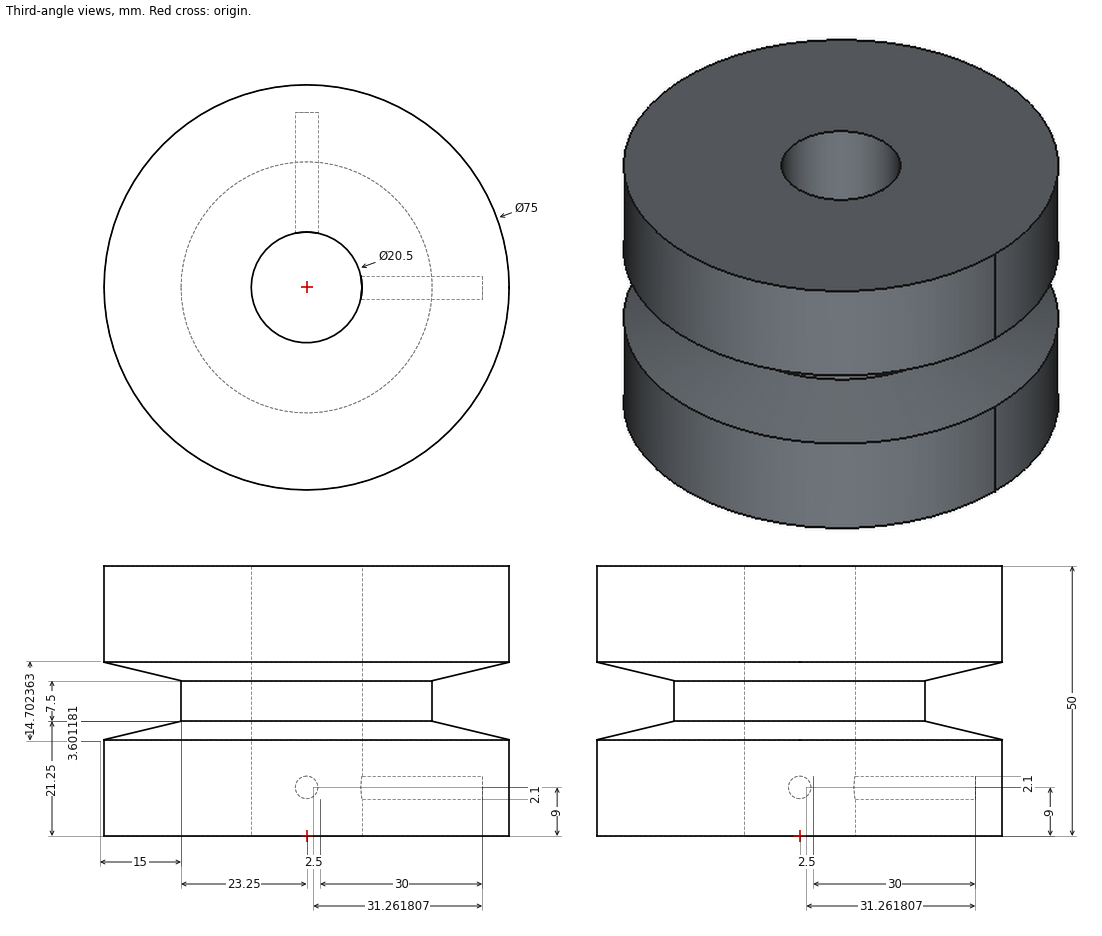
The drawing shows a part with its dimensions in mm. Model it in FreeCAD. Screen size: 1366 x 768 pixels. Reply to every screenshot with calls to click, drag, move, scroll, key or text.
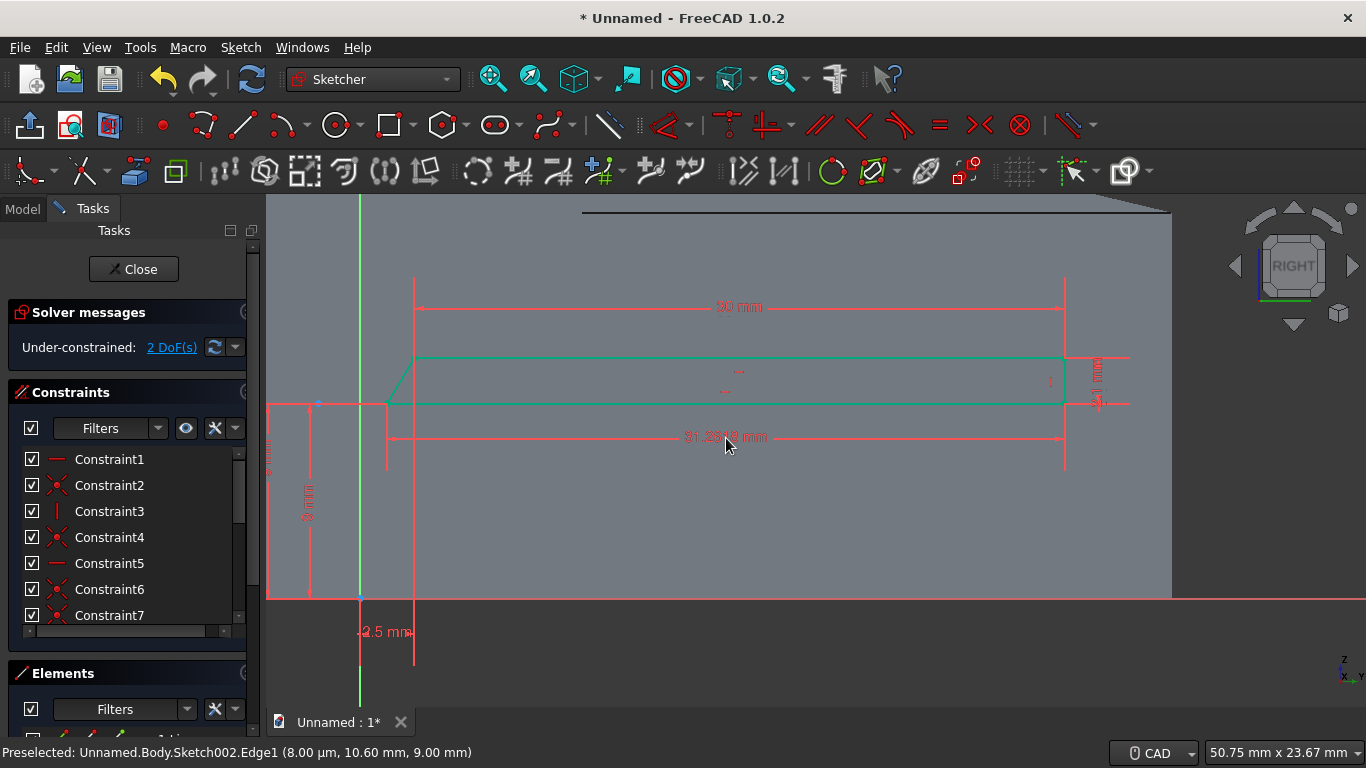
click(134, 269)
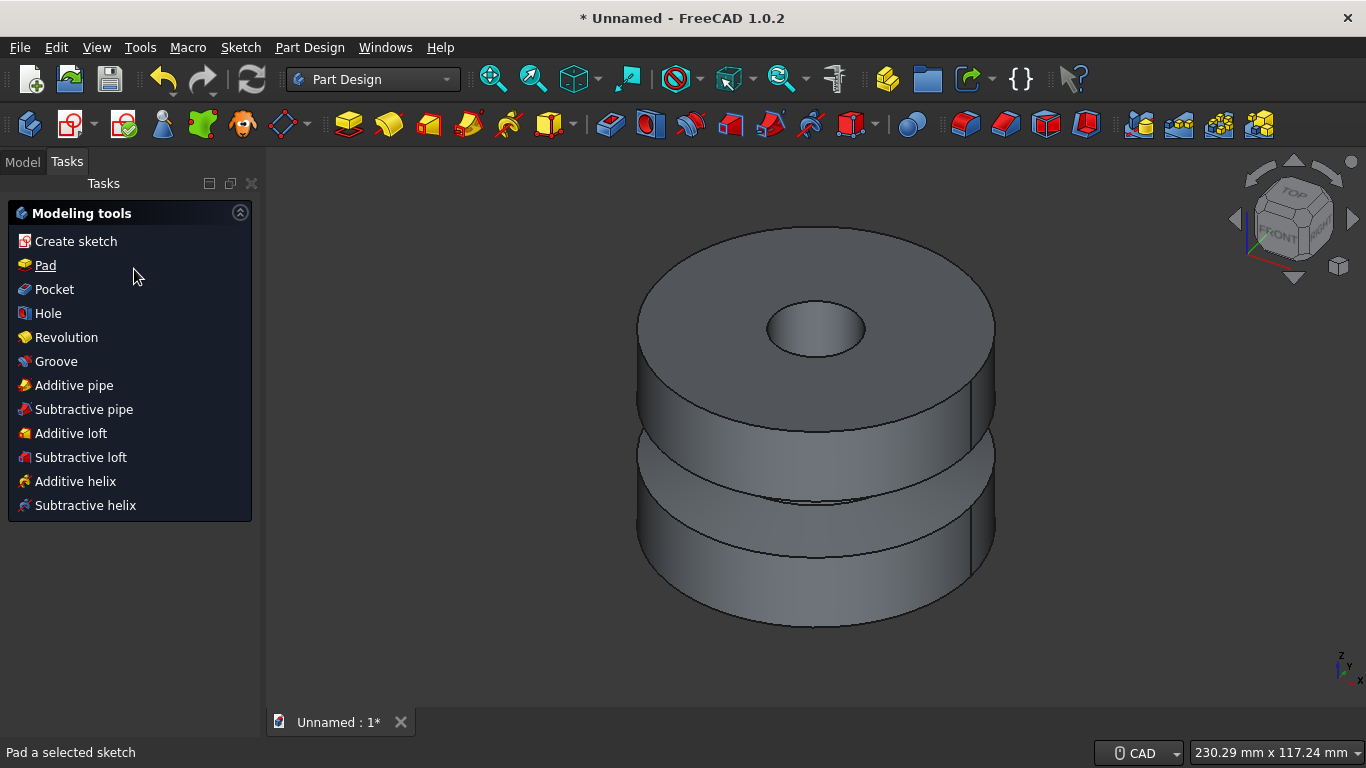
click(692, 124)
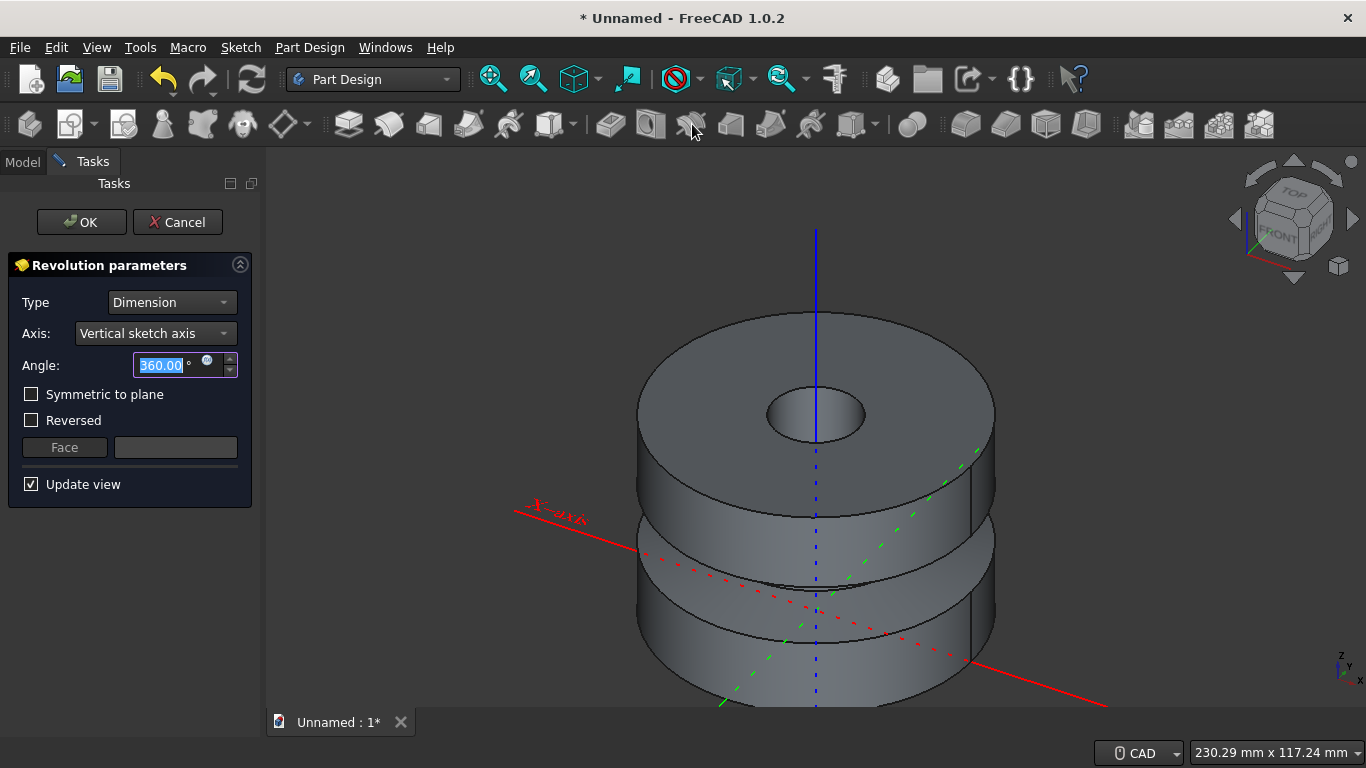
click(156, 334)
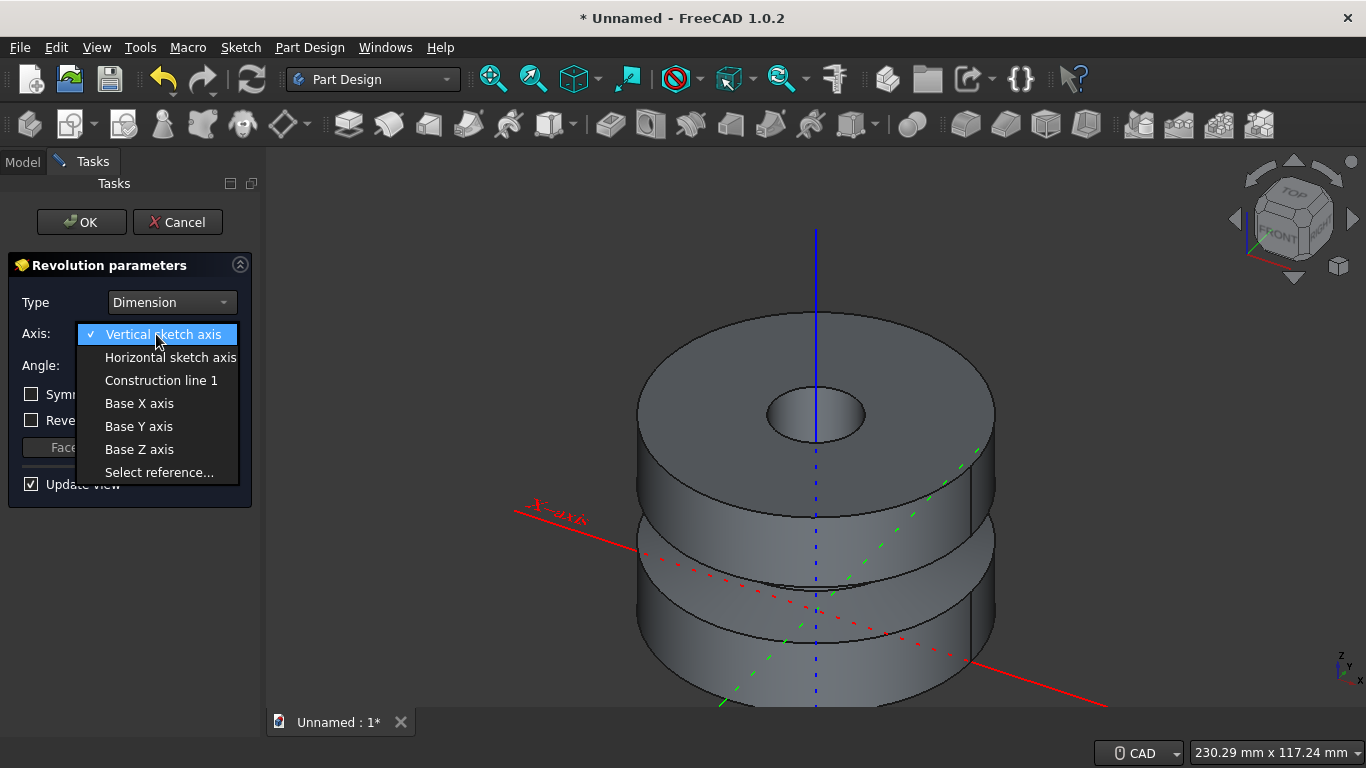
click(156, 380)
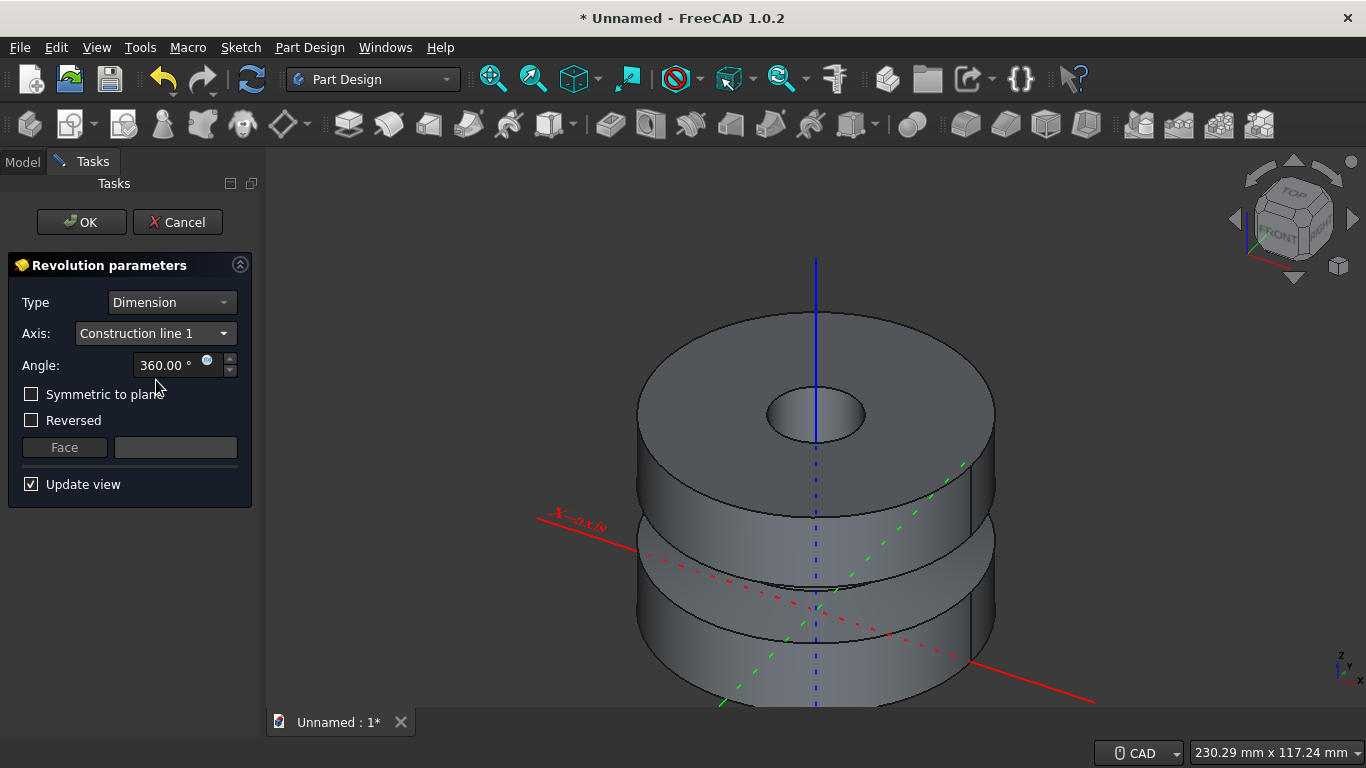
click(82, 222)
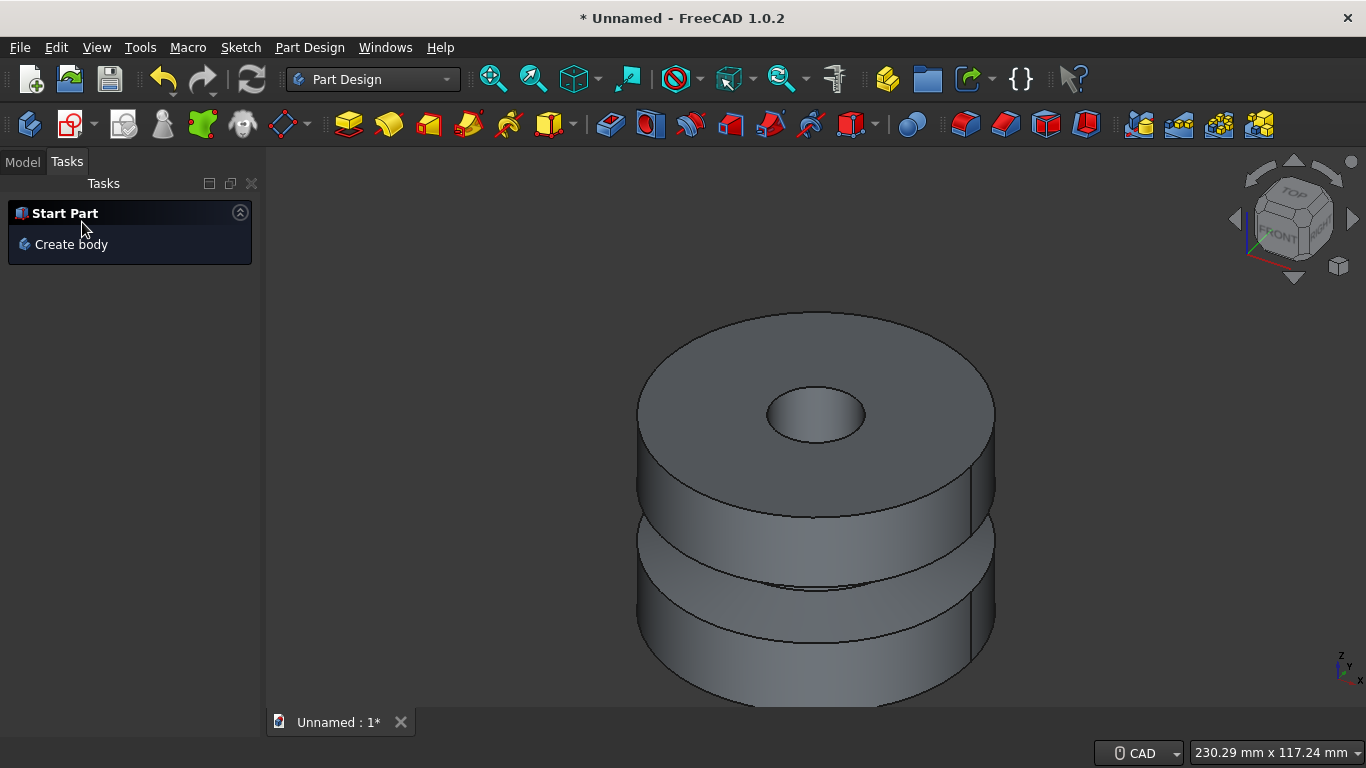
key(v)
key(f)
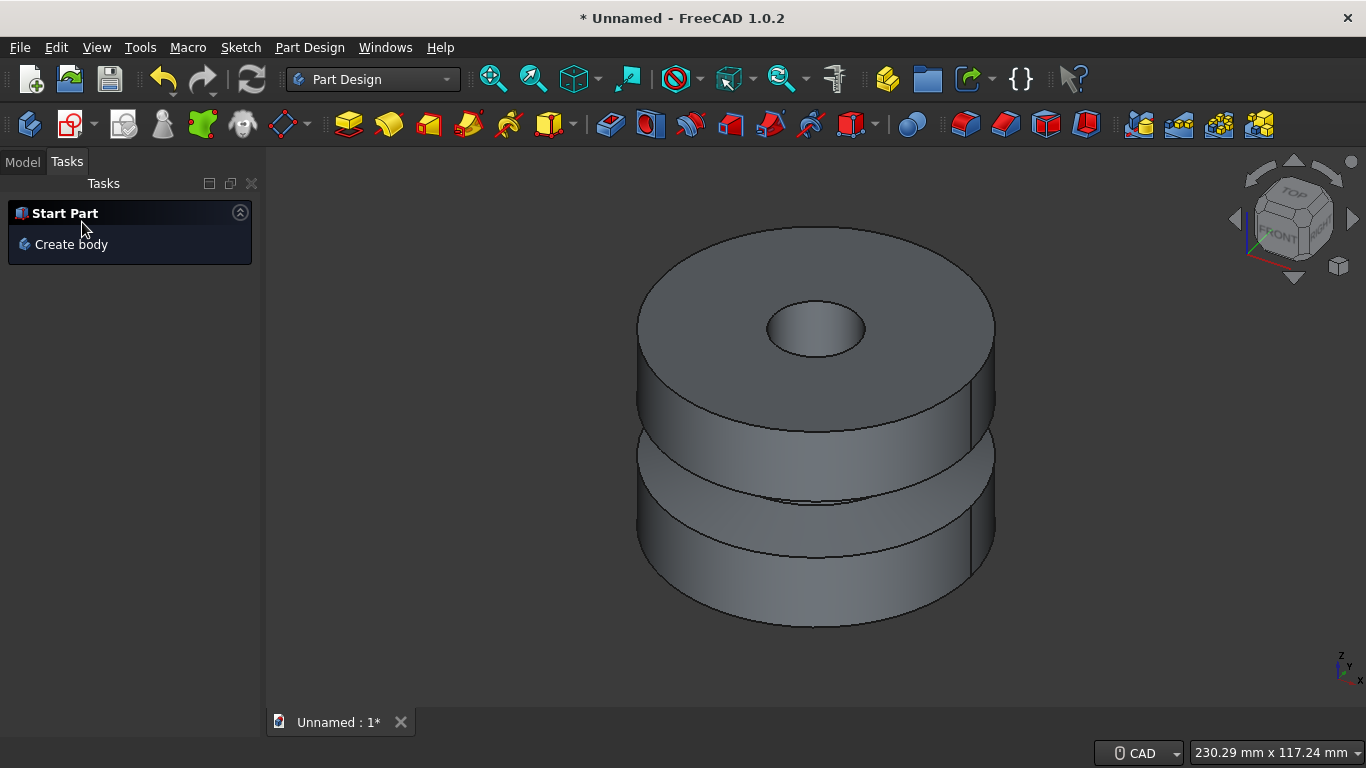
click(70, 124)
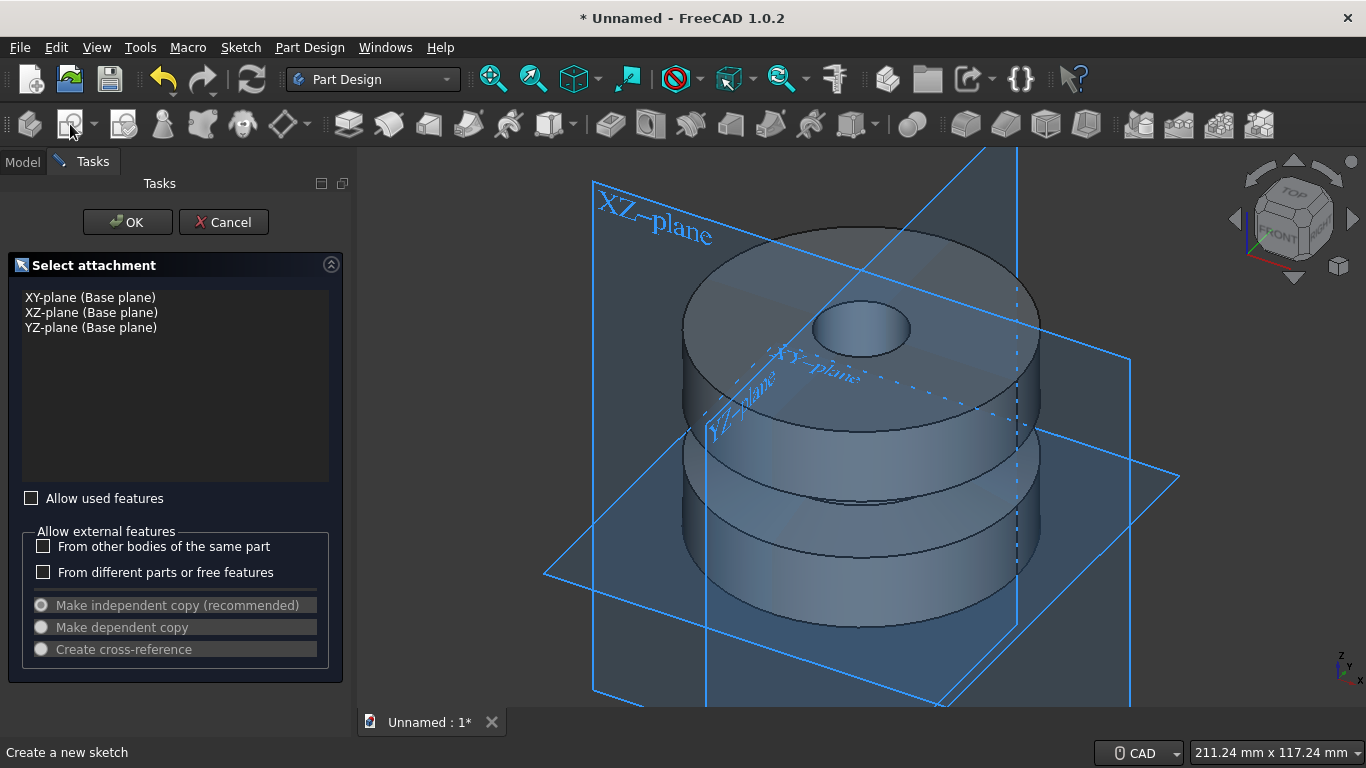
click(82, 312)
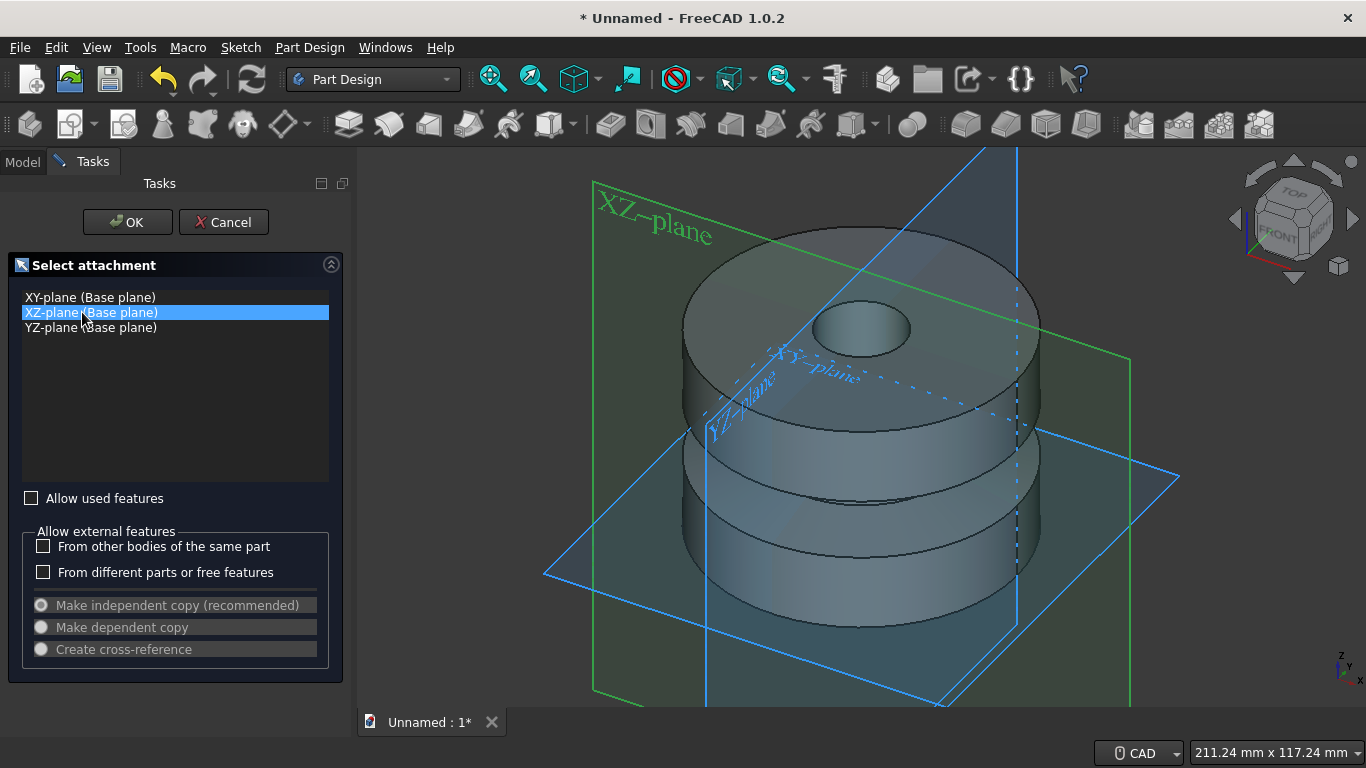
click(128, 222)